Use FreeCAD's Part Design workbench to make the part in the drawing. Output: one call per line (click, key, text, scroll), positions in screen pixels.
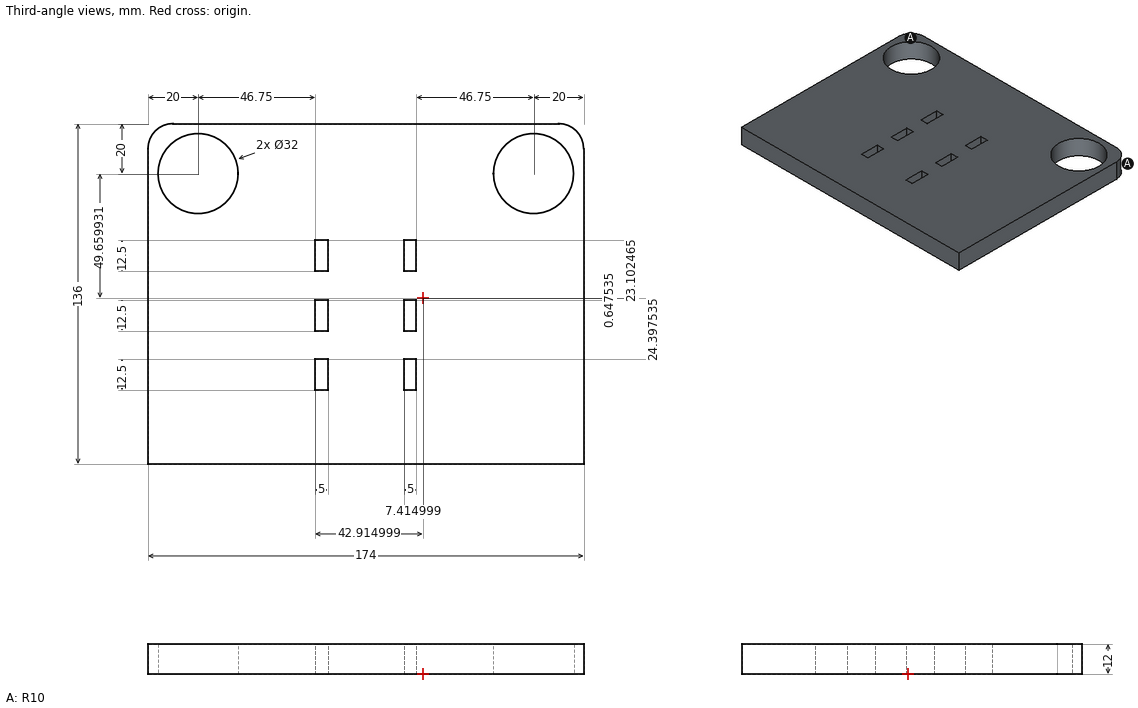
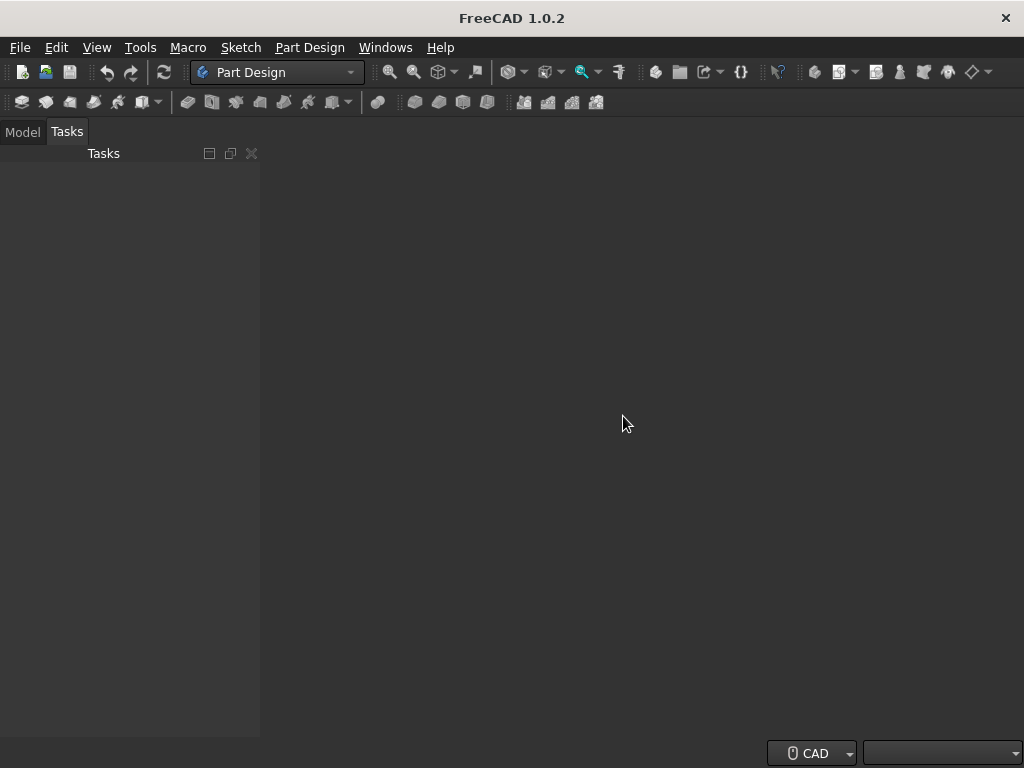
key(ctrl+n)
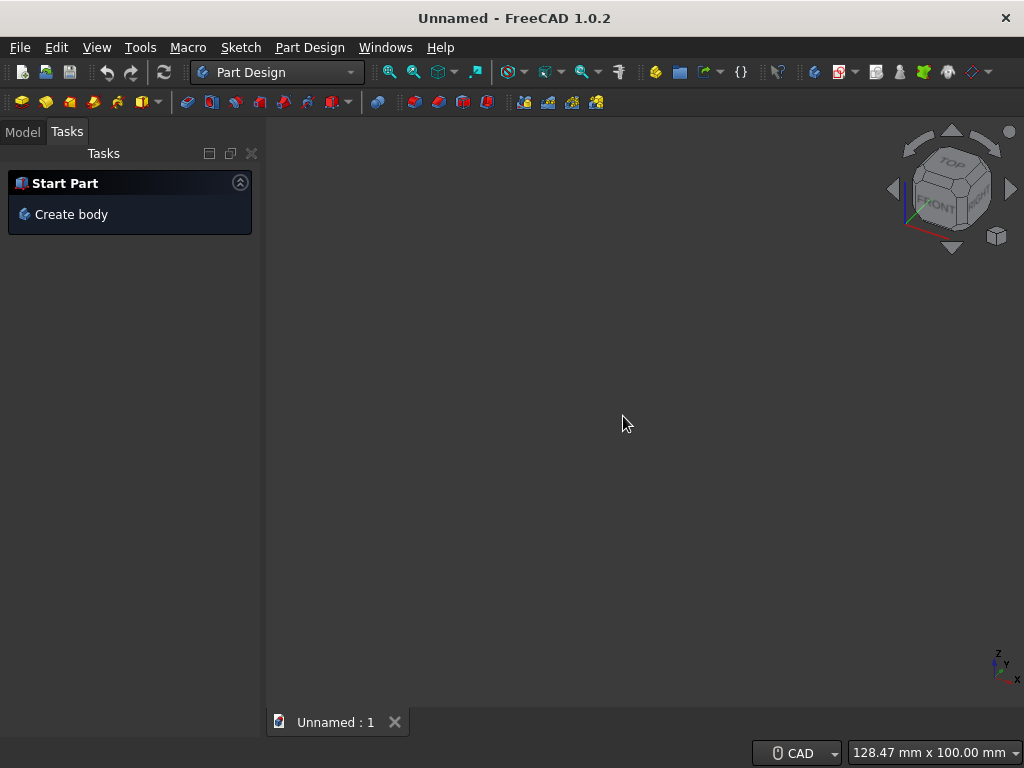
click(840, 72)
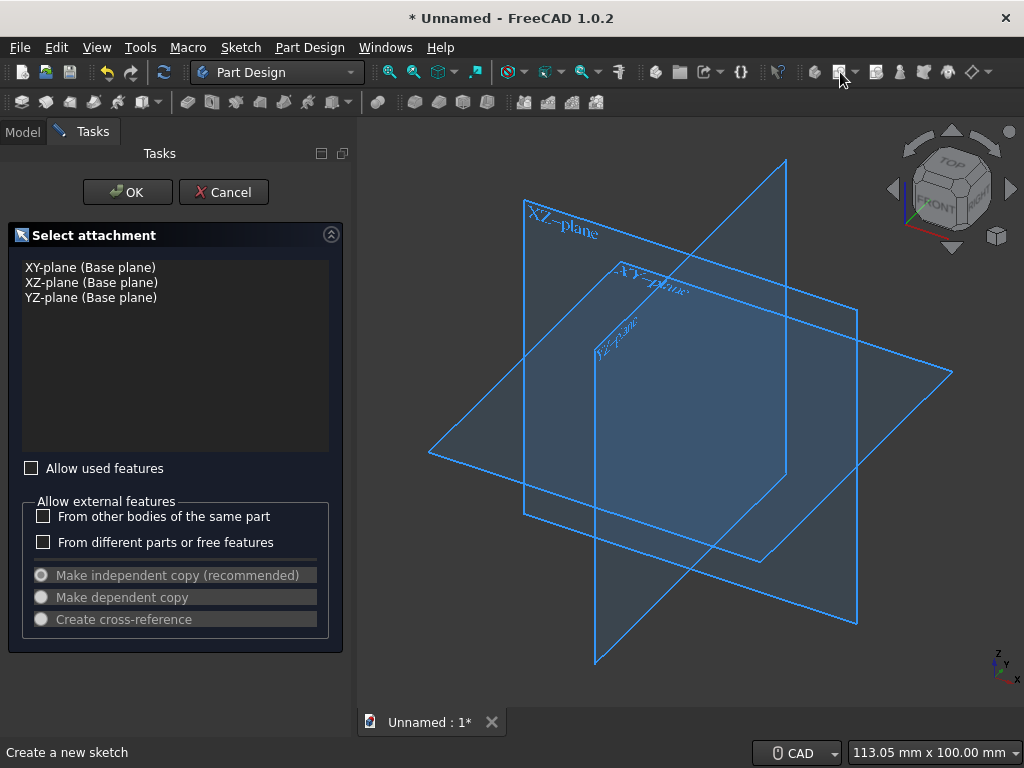
click(82, 268)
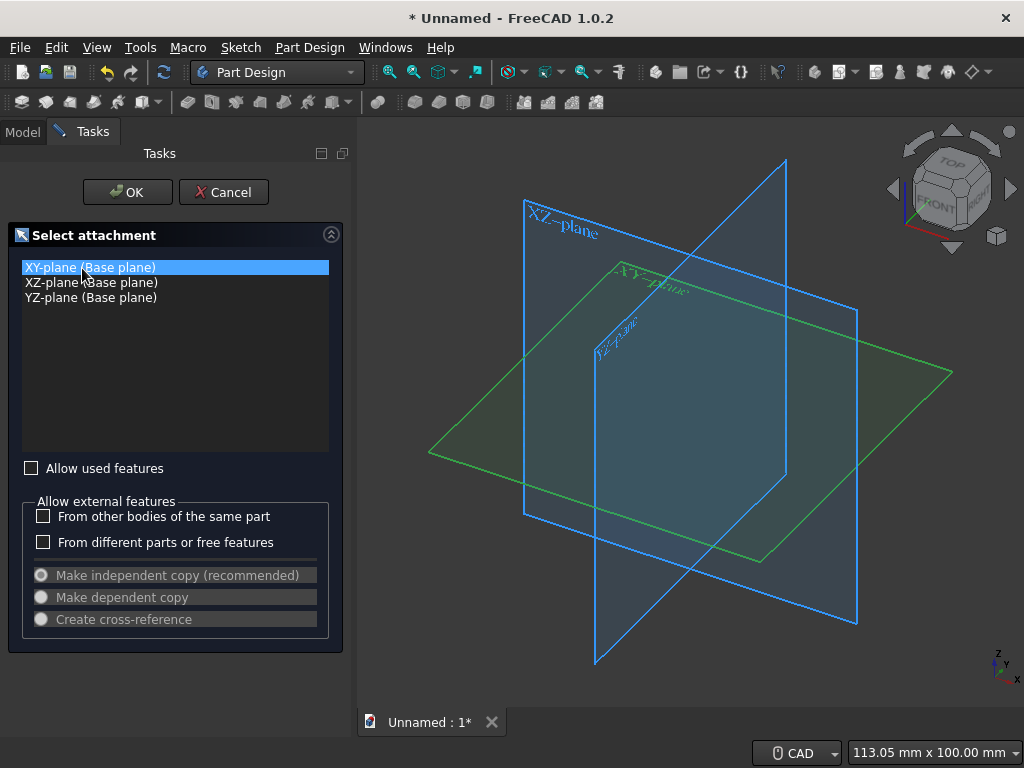
click(128, 192)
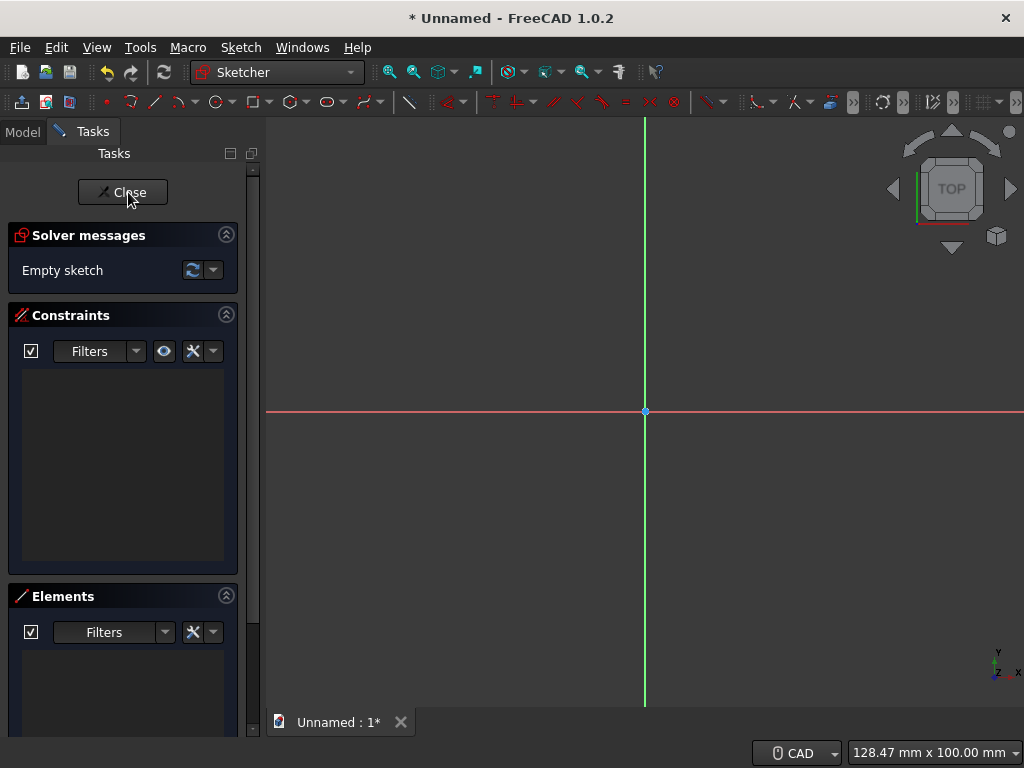
scroll(614, 418, down, 5)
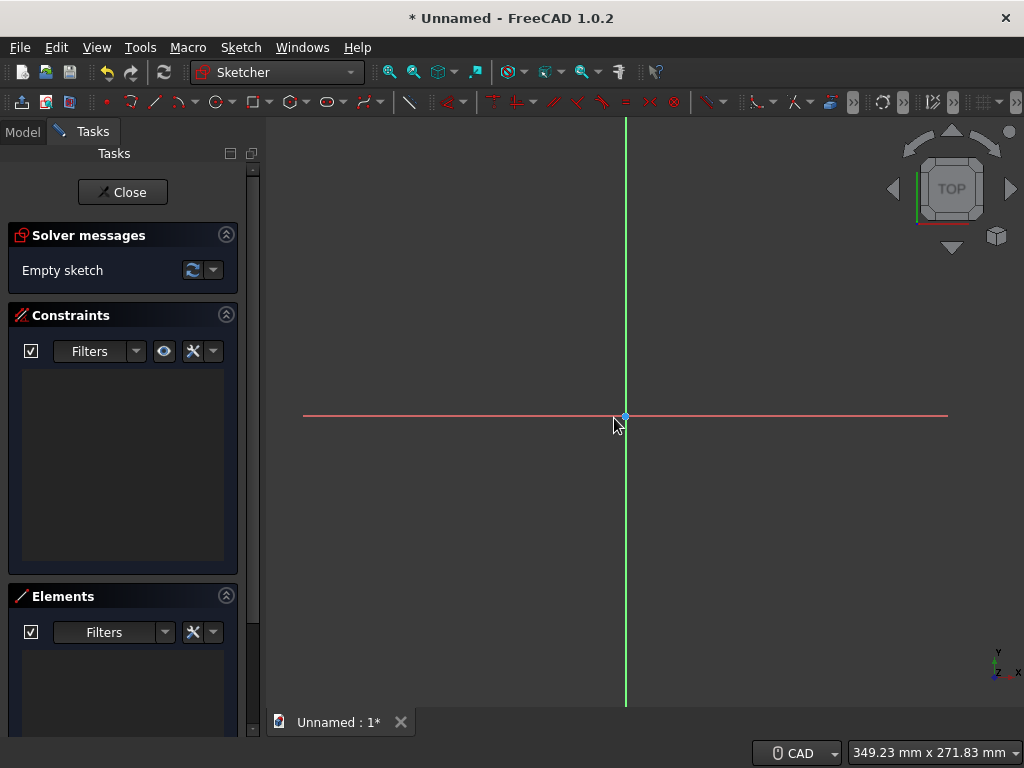
click(254, 102)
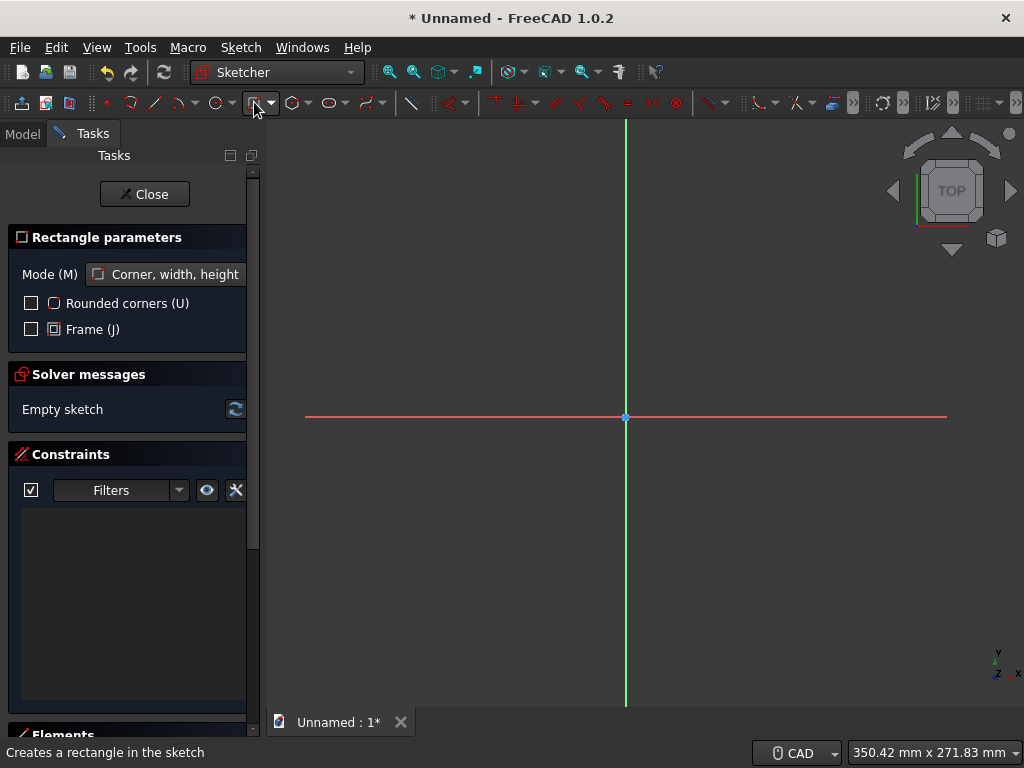
click(389, 266)
click(765, 561)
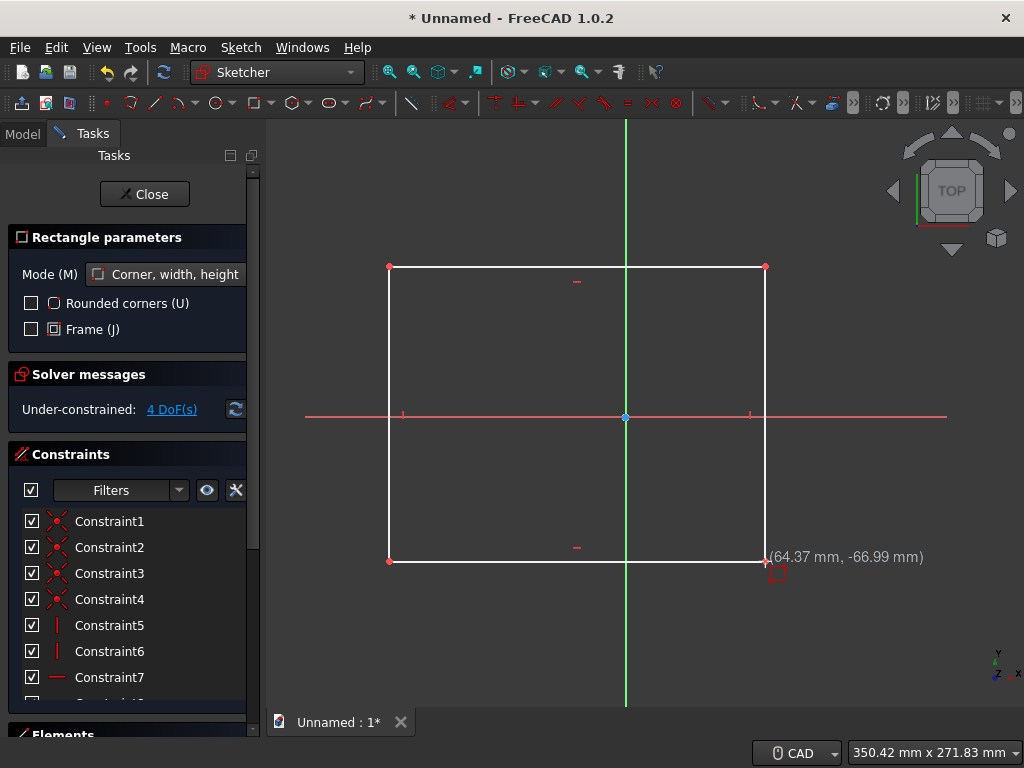
scroll(533, 470, up, 2)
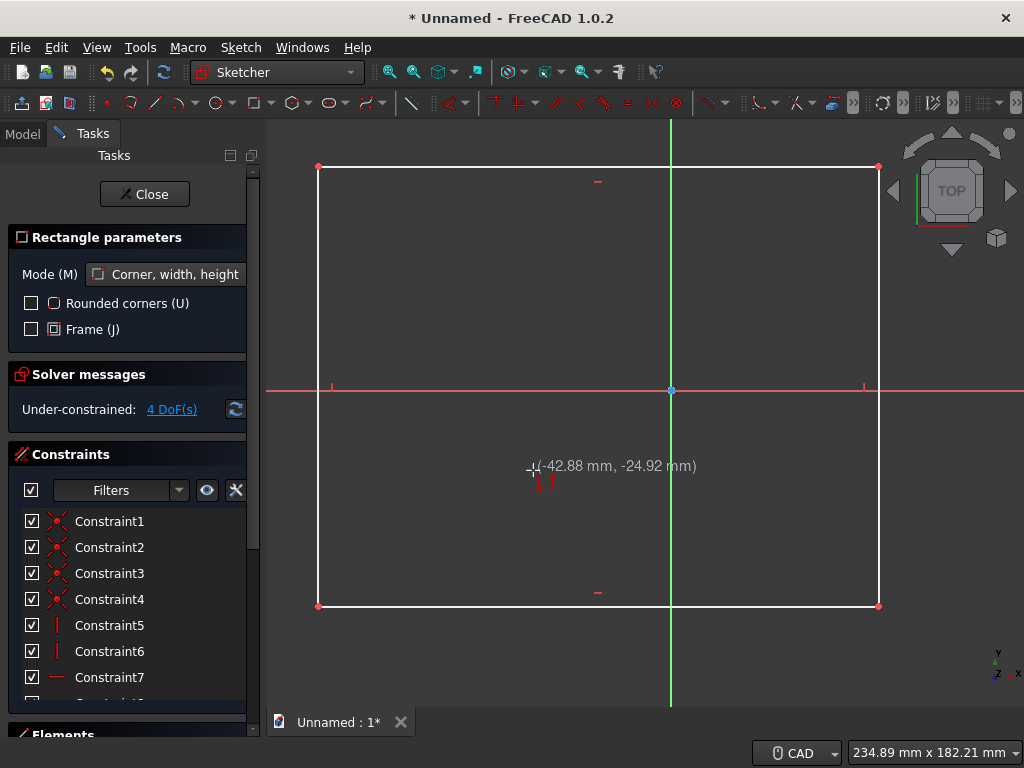
click(533, 470)
click(549, 510)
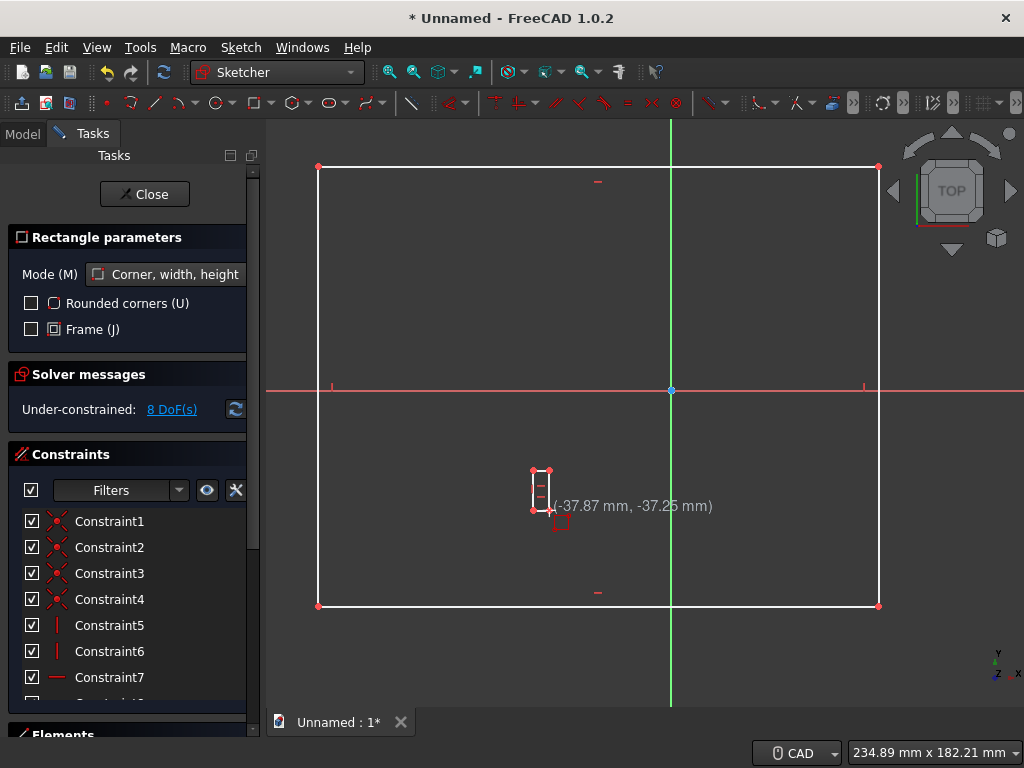
scroll(533, 393, up, 11)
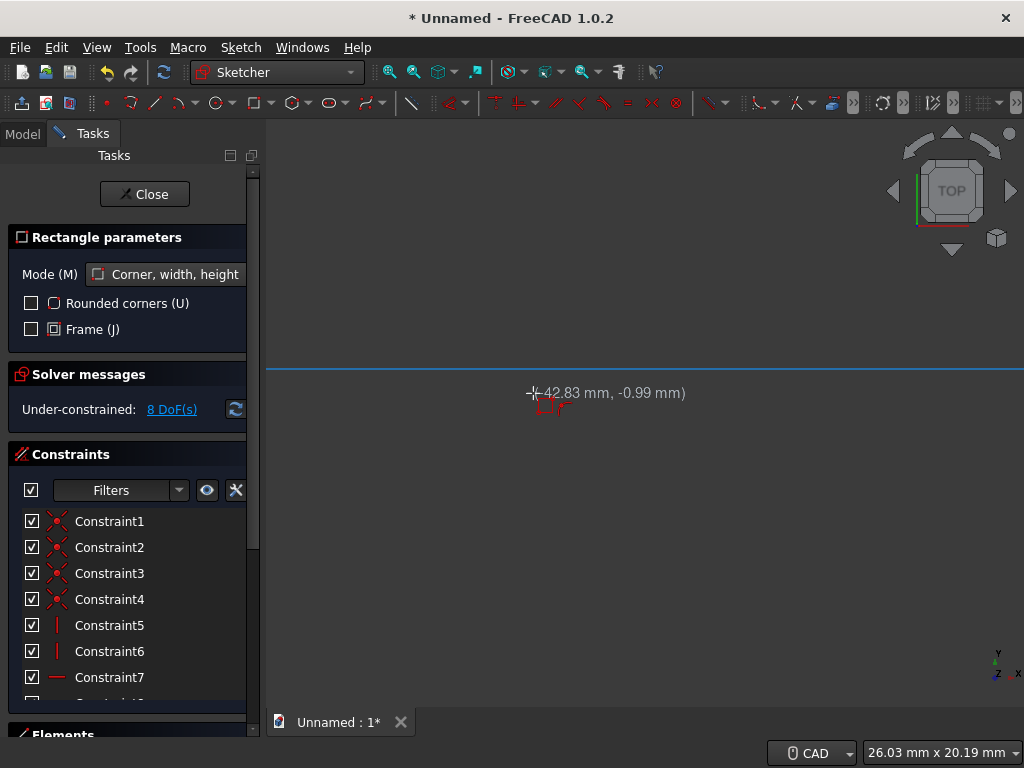
click(528, 388)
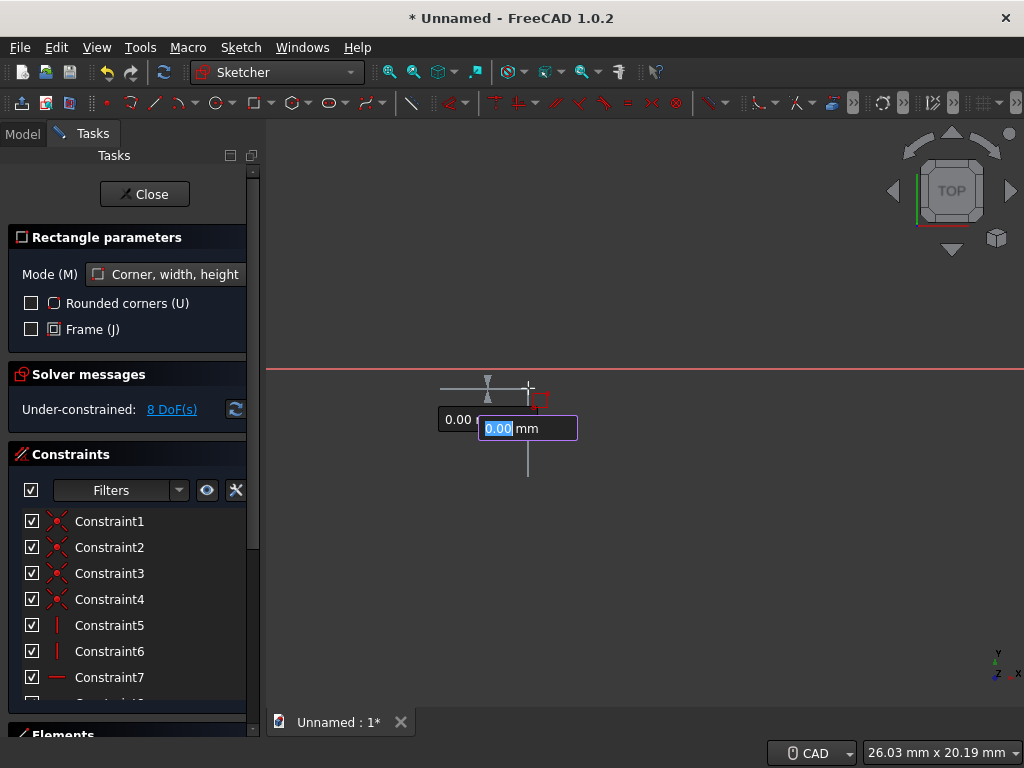
scroll(533, 420, down, 13)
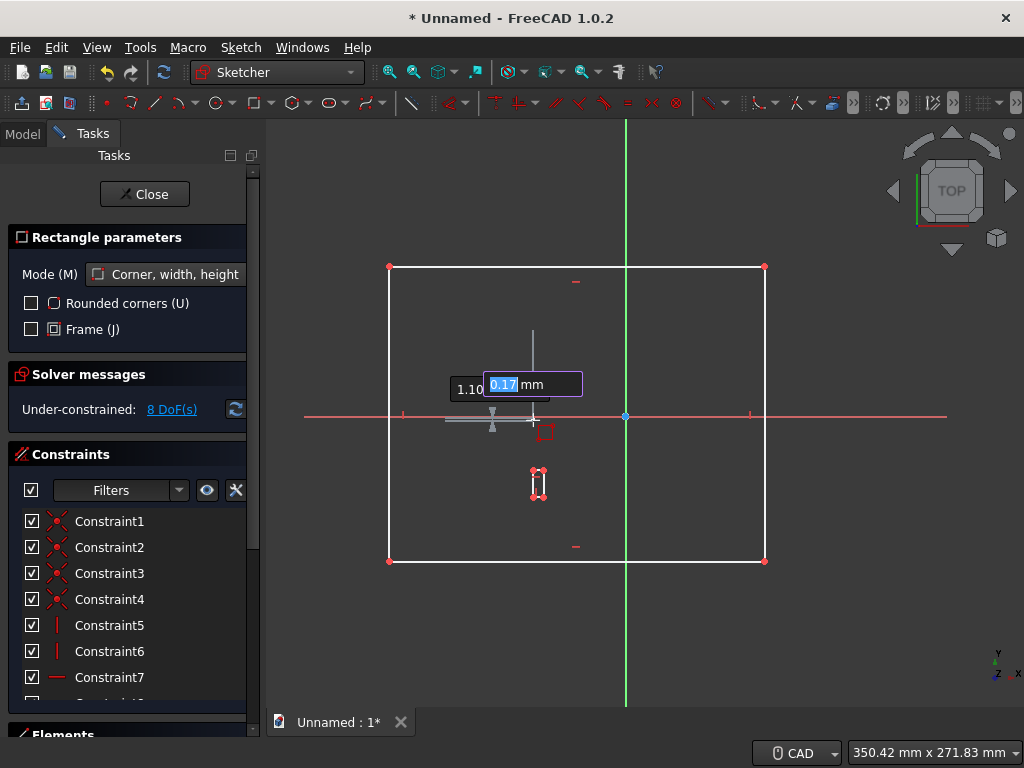
click(544, 445)